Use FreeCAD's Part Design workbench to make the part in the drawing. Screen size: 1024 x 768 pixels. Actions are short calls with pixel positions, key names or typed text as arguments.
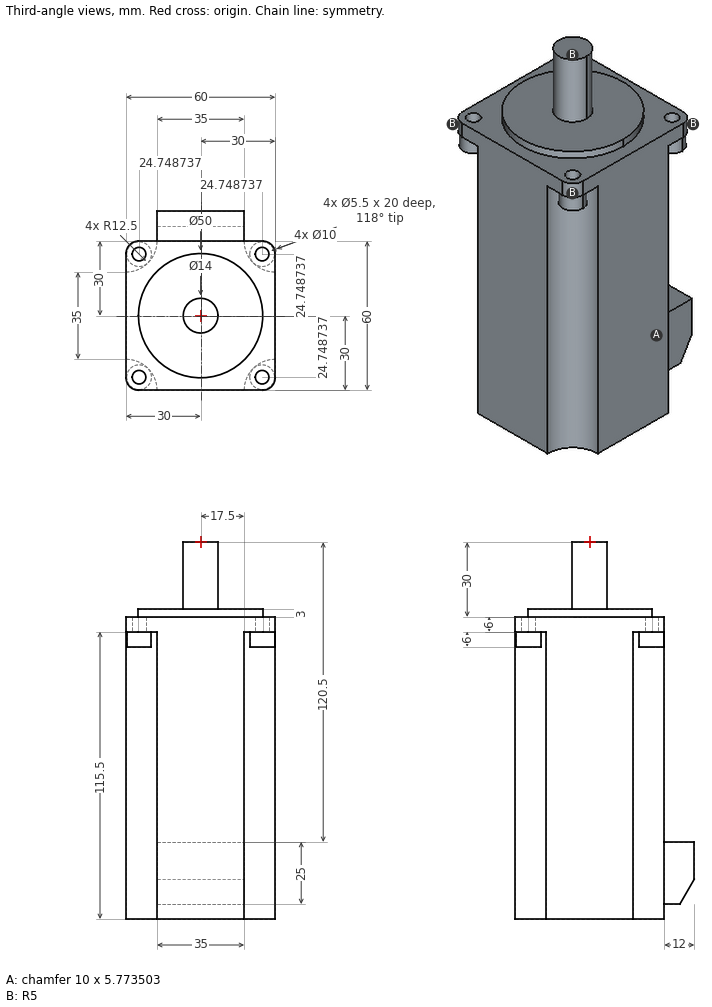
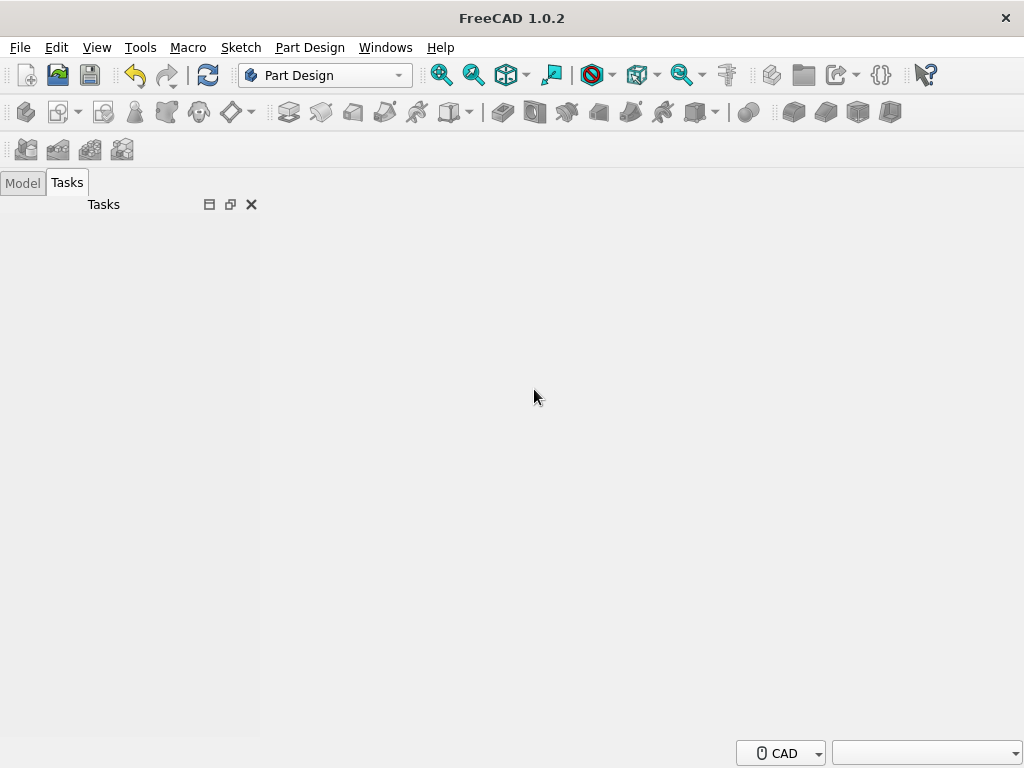
click(26, 76)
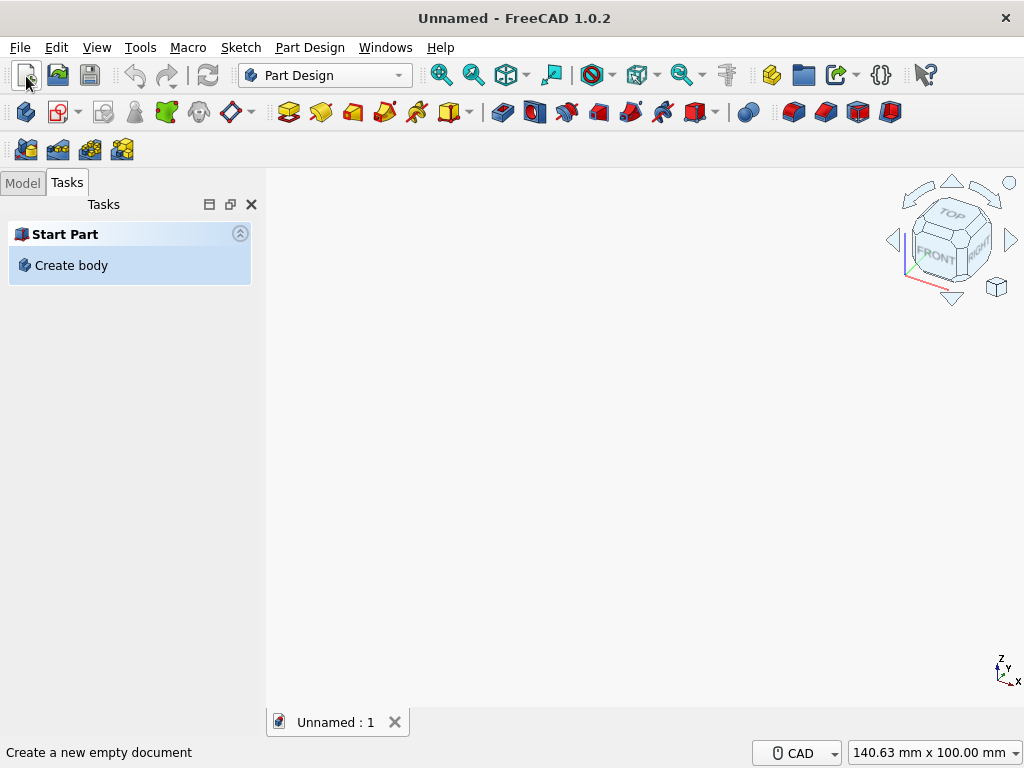
click(58, 112)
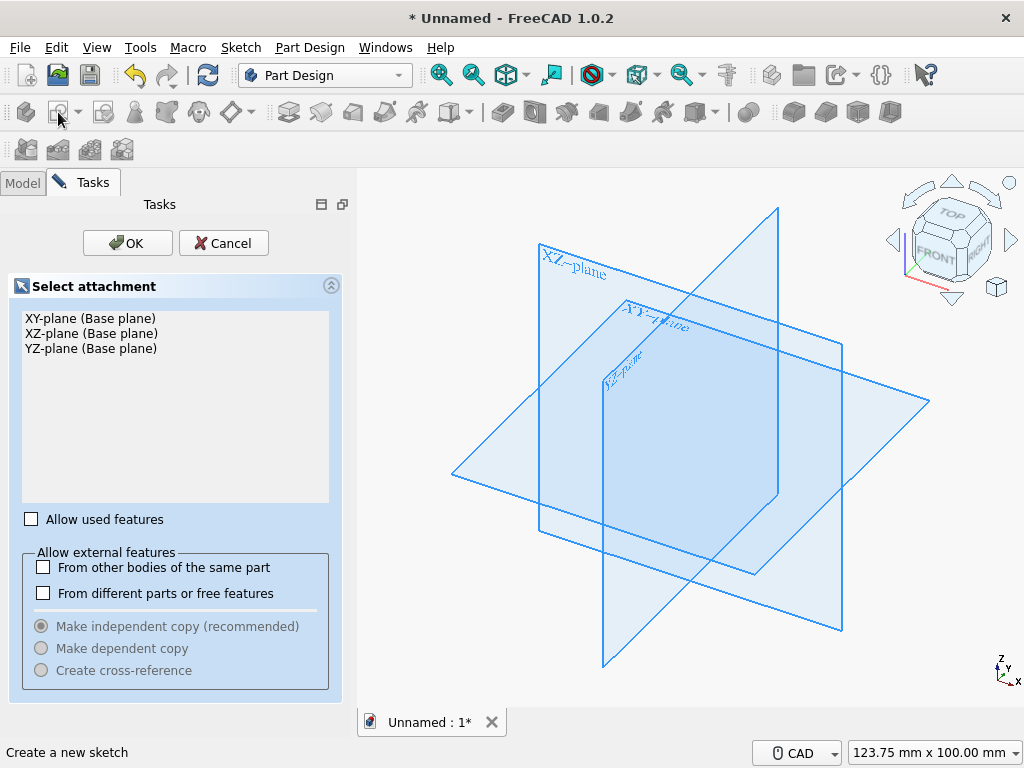
click(82, 318)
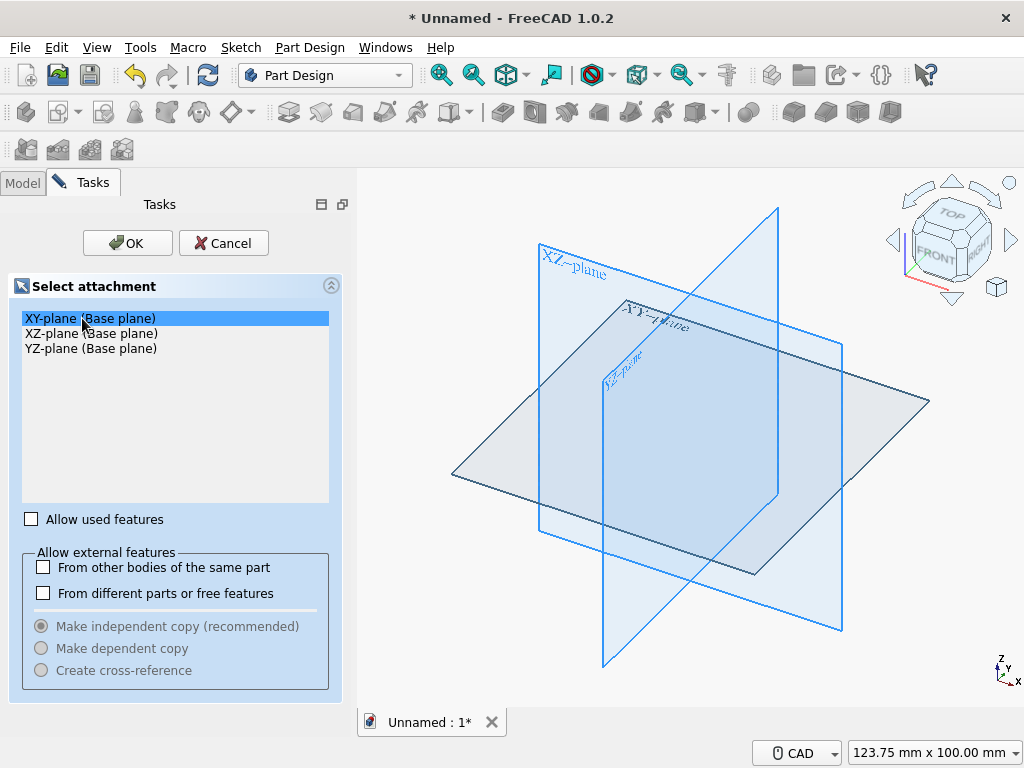
click(128, 243)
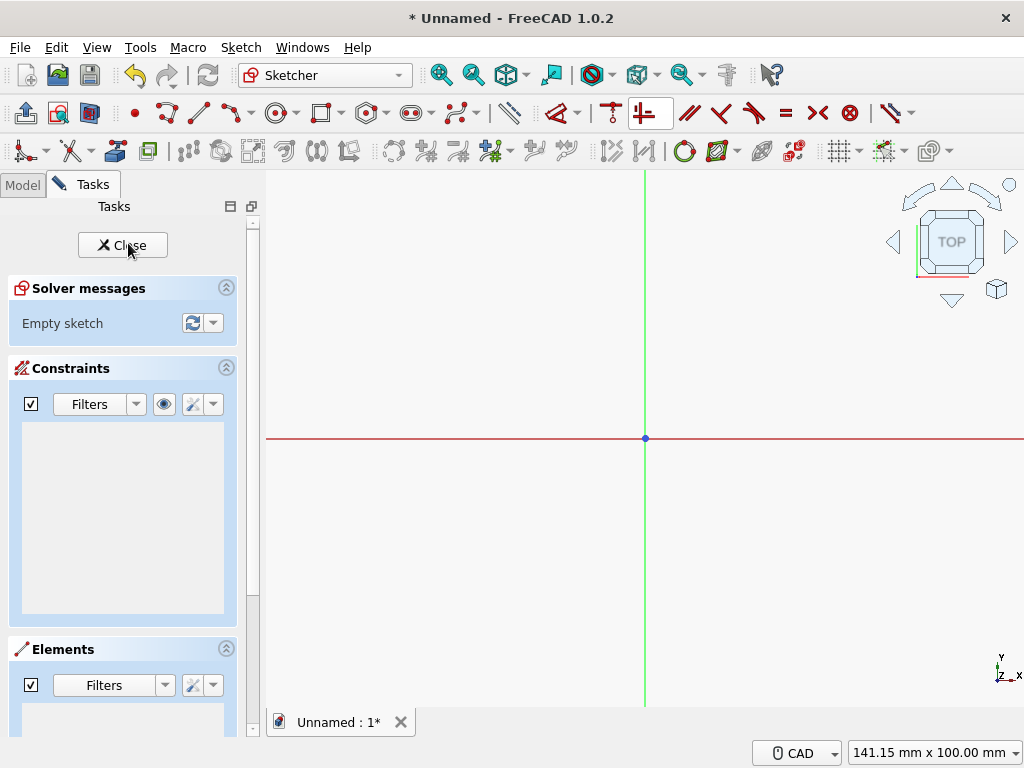
scroll(662, 438, up, 8)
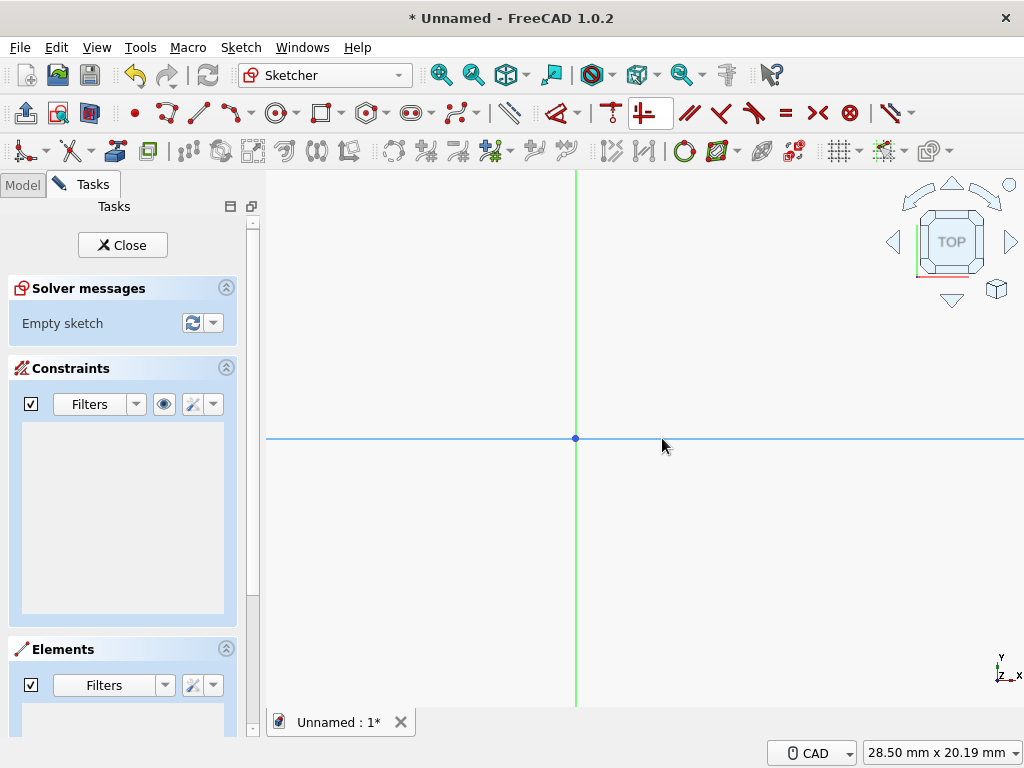
click(276, 114)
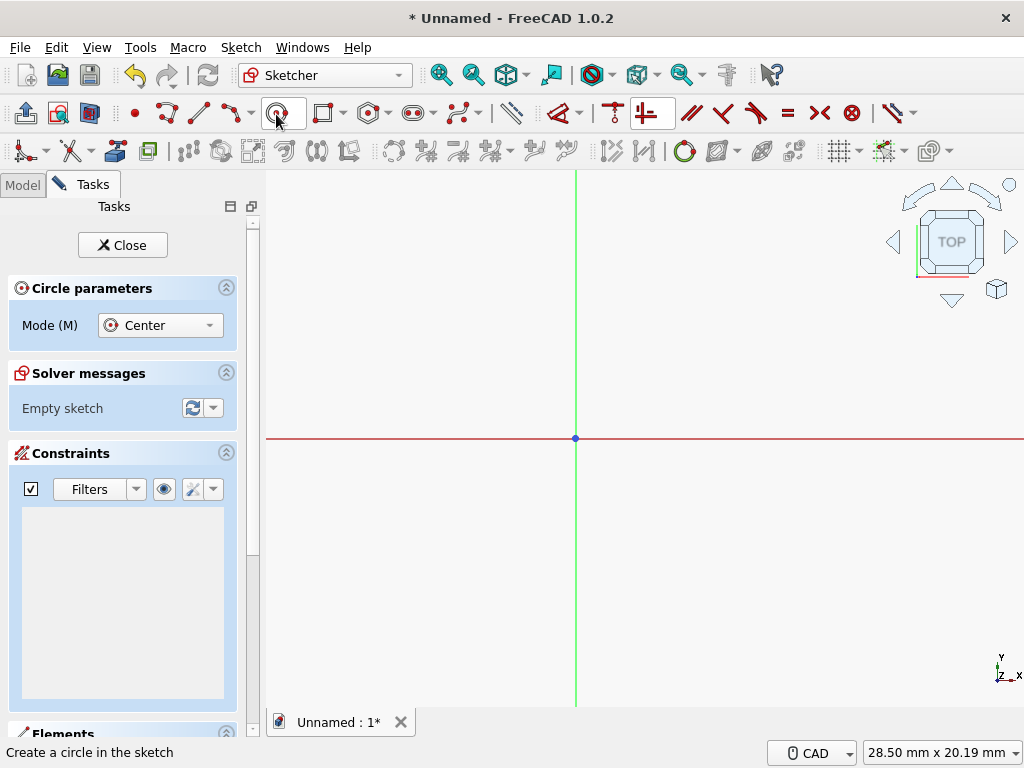
click(576, 438)
click(707, 307)
key(Escape)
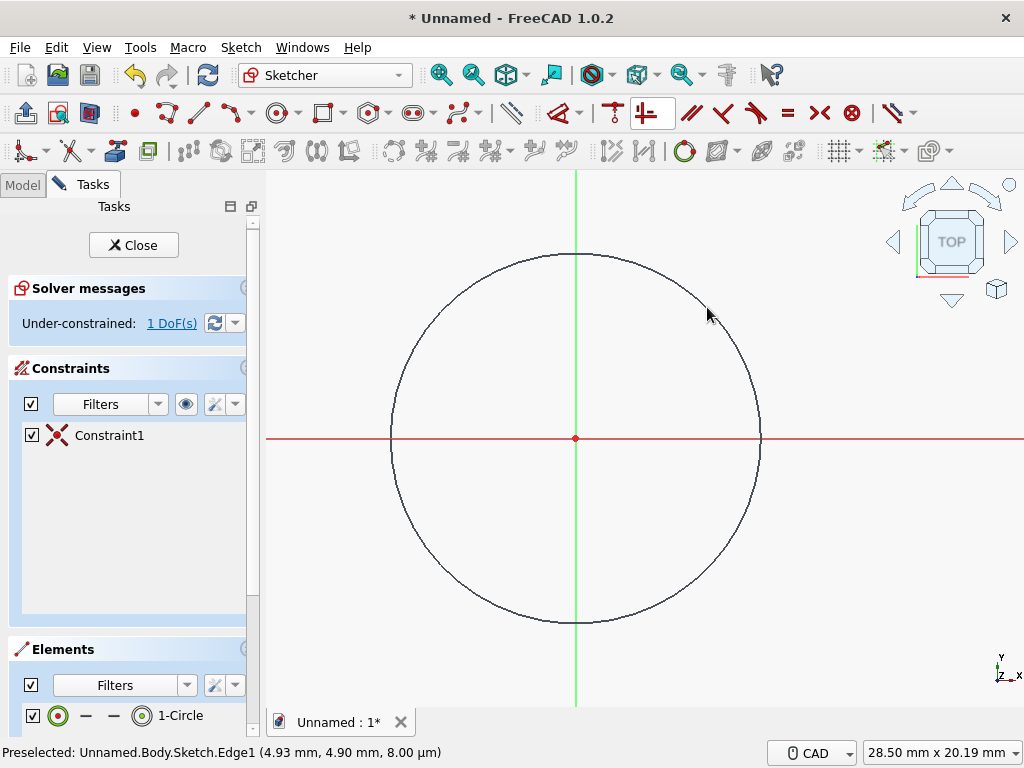
click(558, 114)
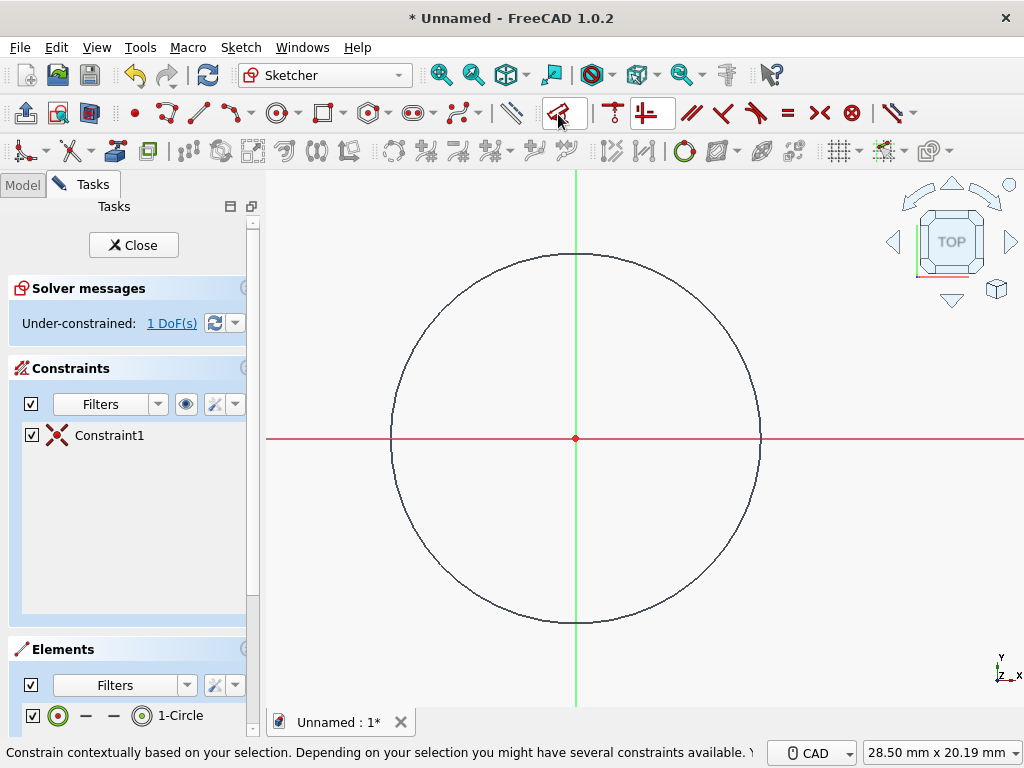
click(706, 307)
click(729, 284)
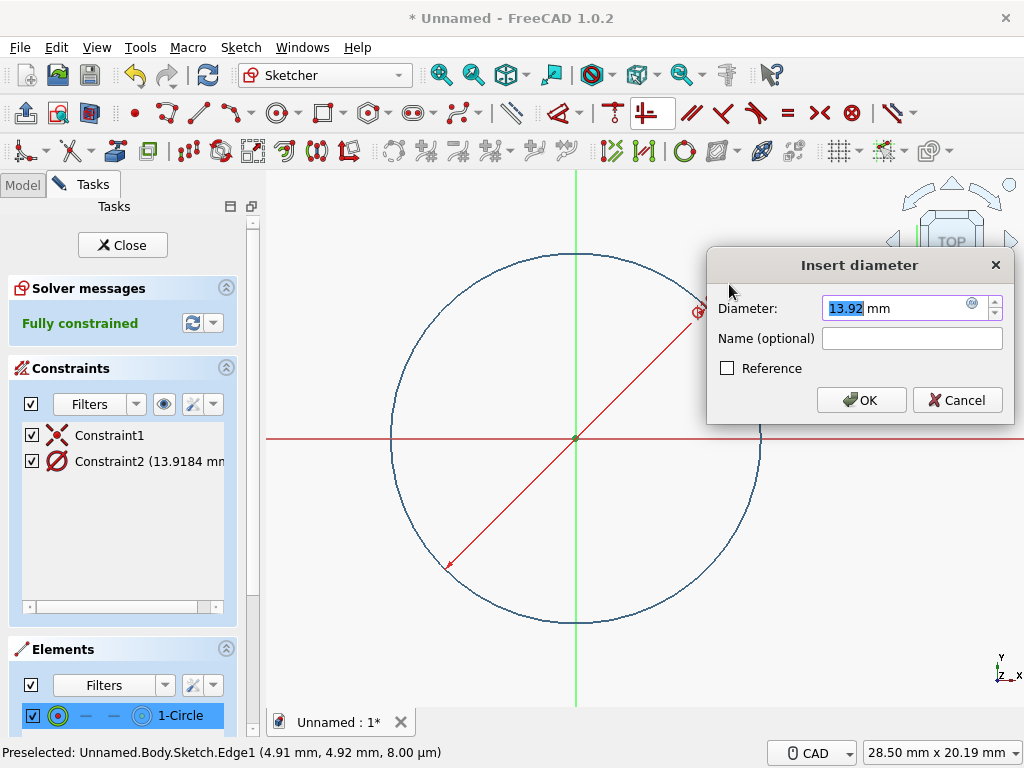
text(14)
key(Return)
key(Escape)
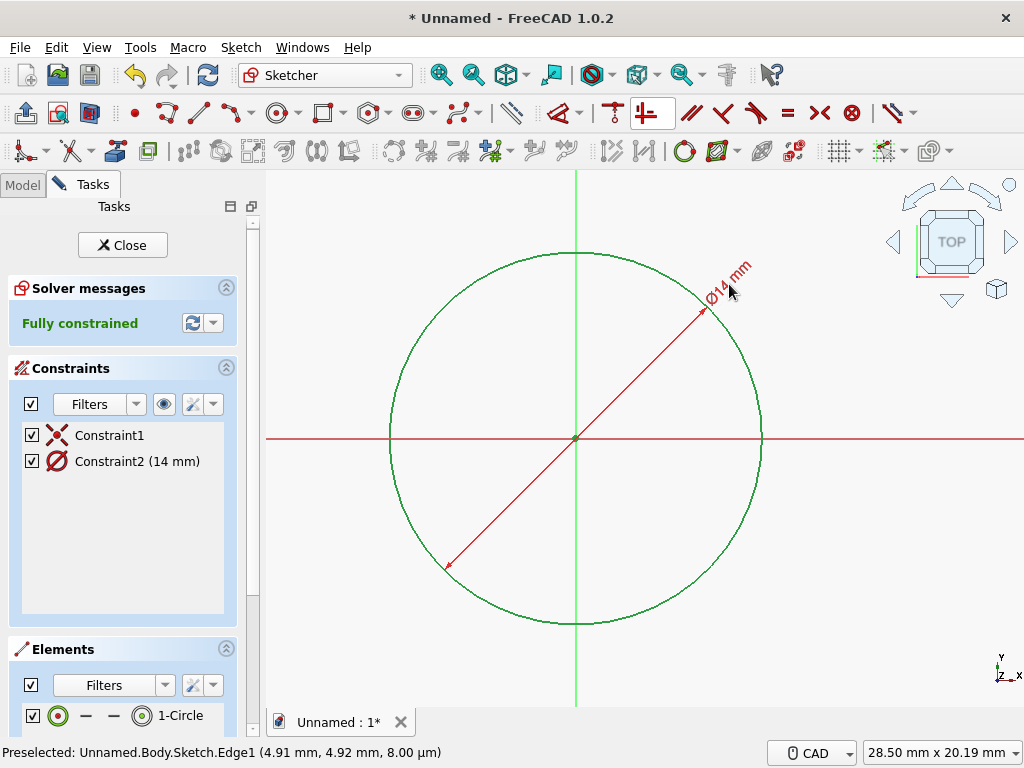
click(123, 245)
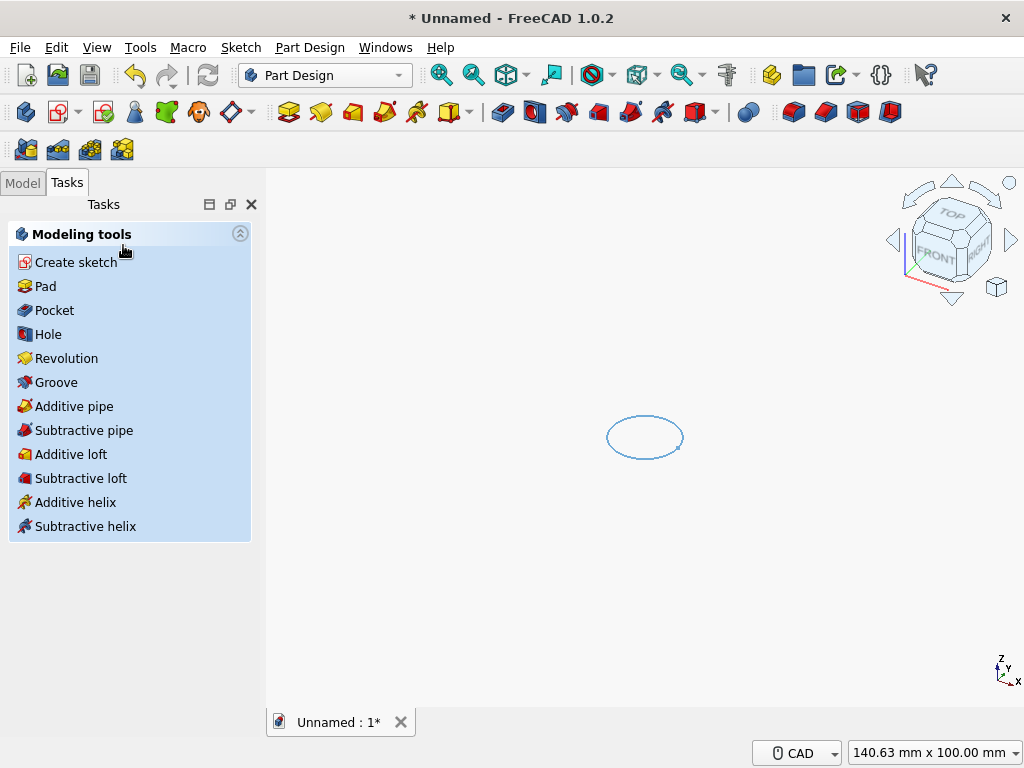
click(290, 112)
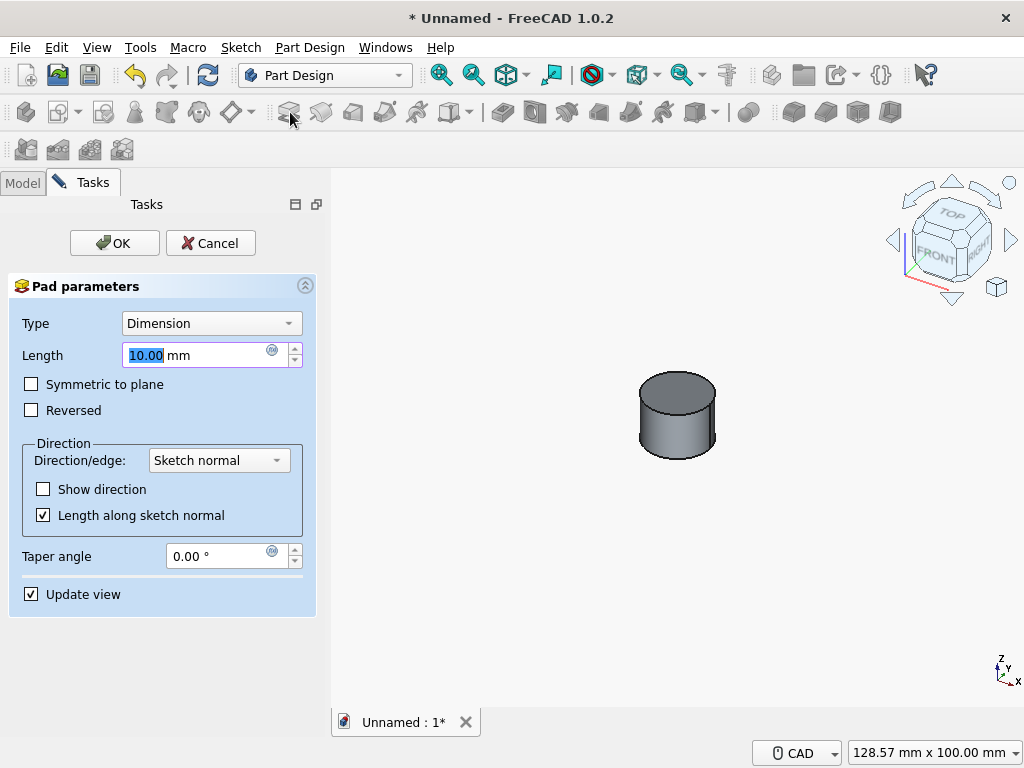
text(30)
key(Tab)